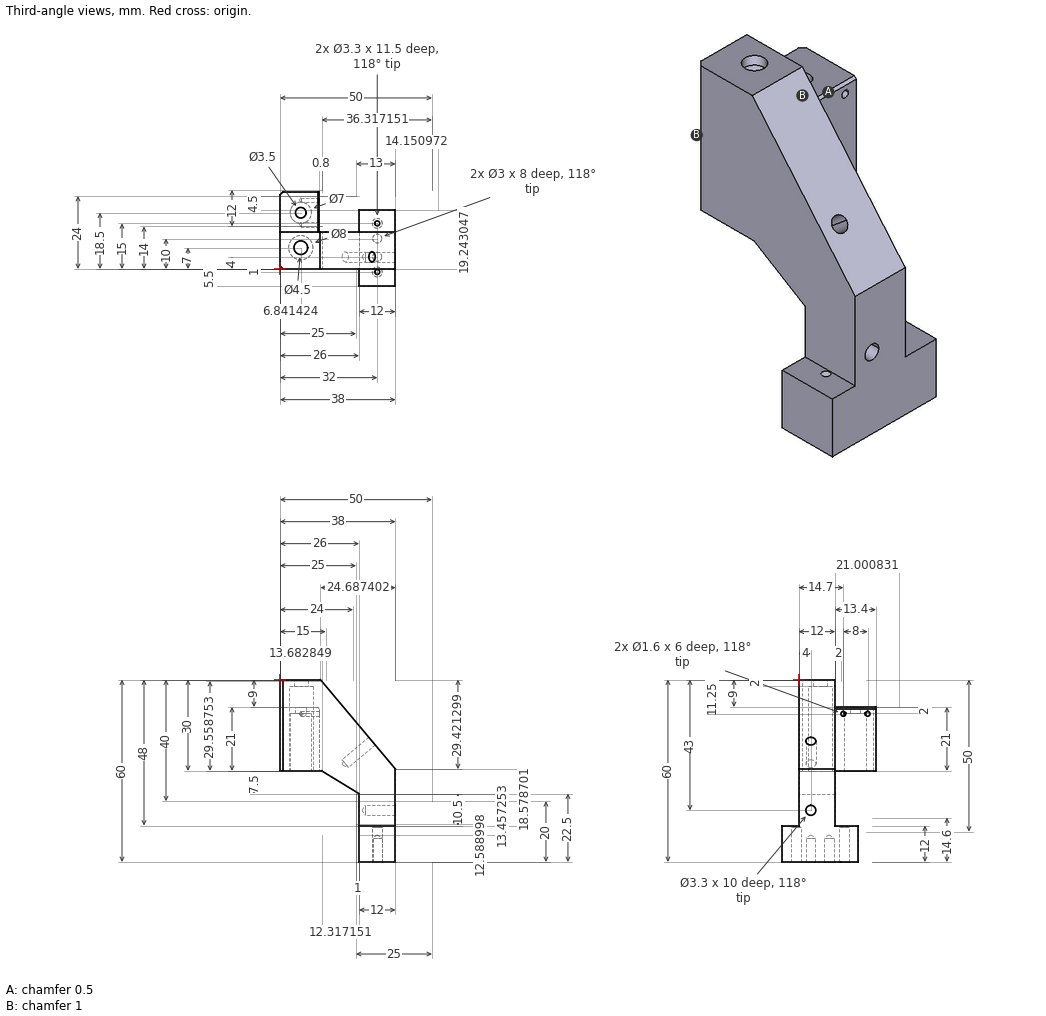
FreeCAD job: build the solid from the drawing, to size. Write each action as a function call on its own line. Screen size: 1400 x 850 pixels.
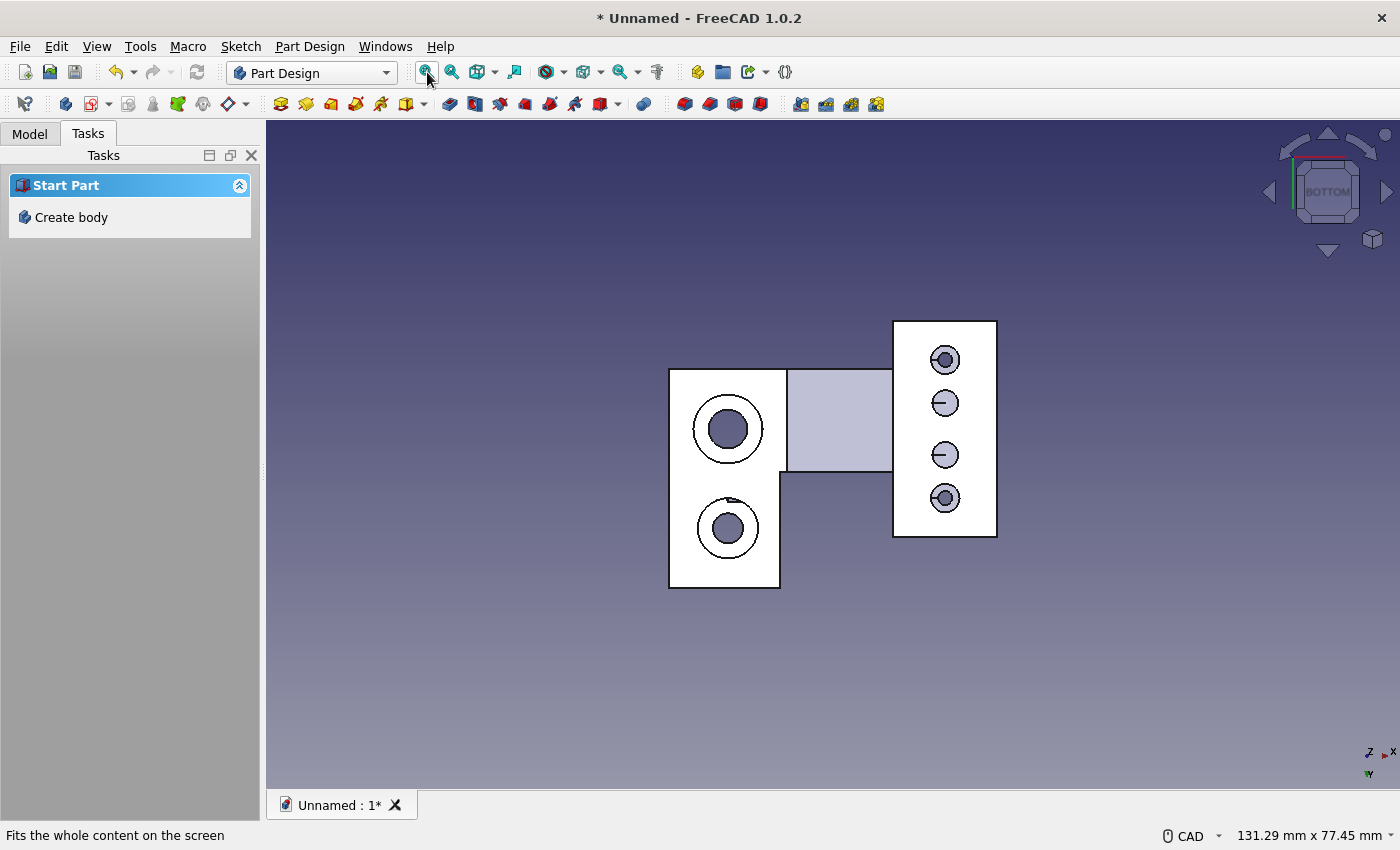
key(0)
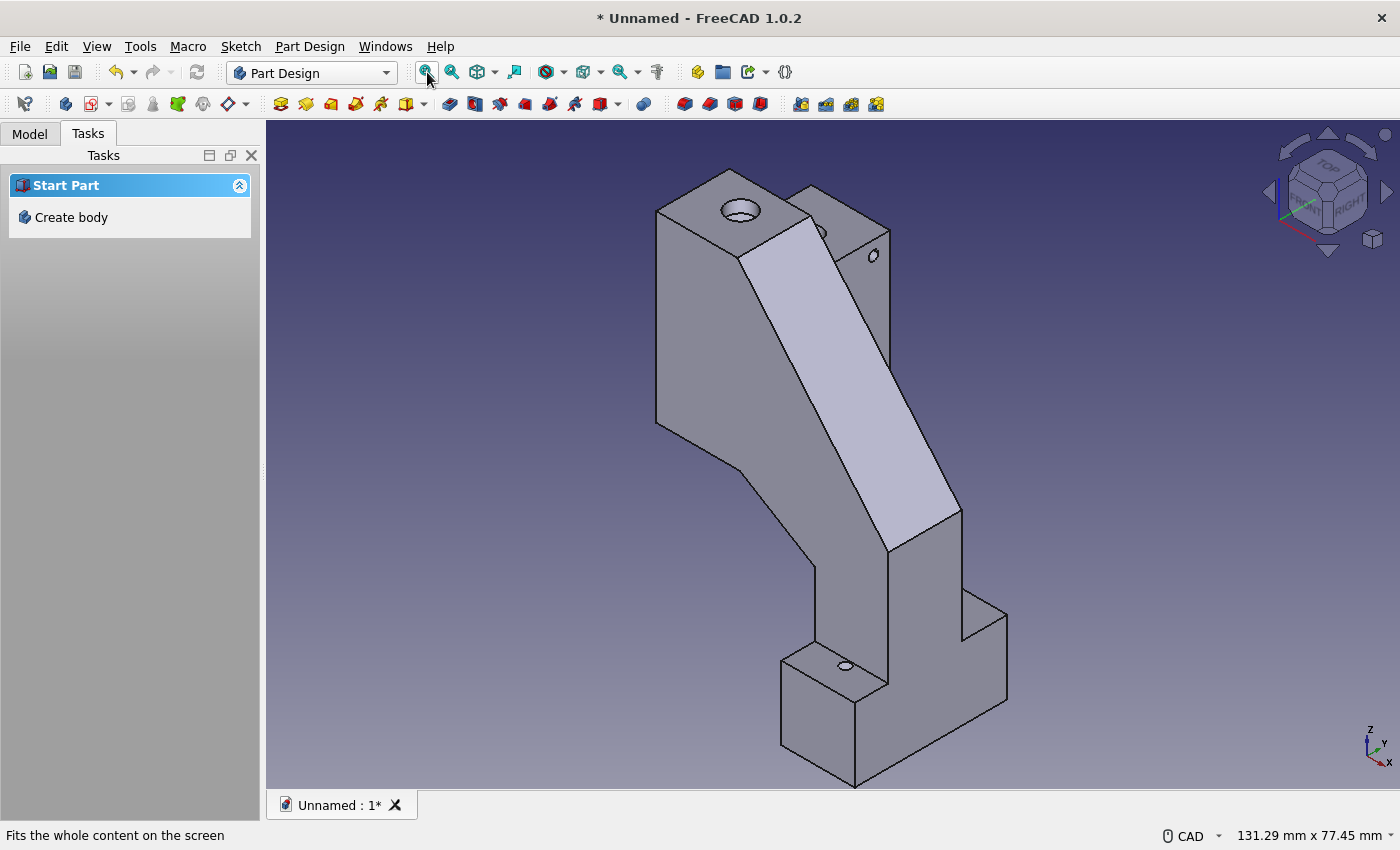
click(849, 253)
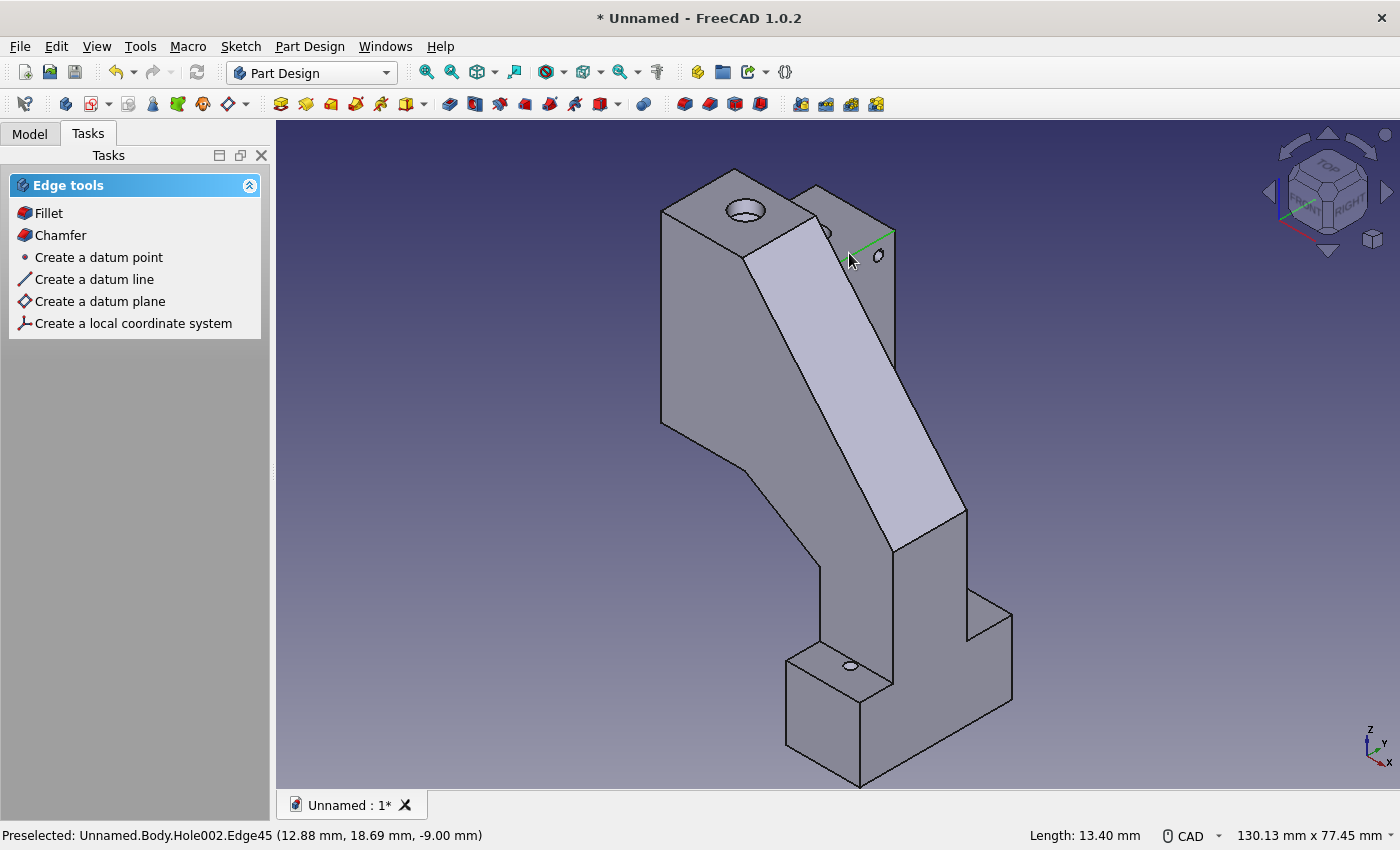
click(710, 104)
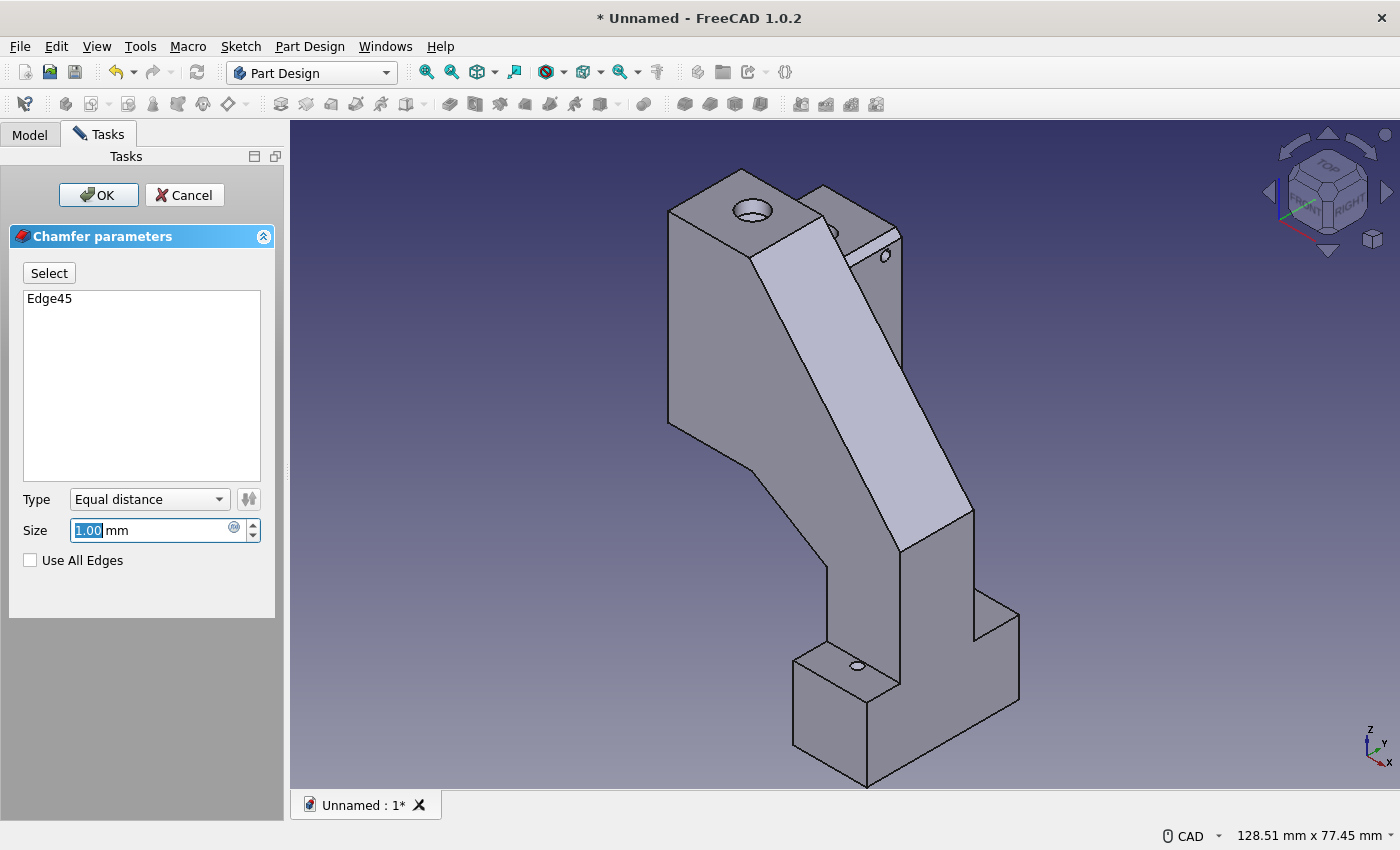
text(0.5)
key(Tab)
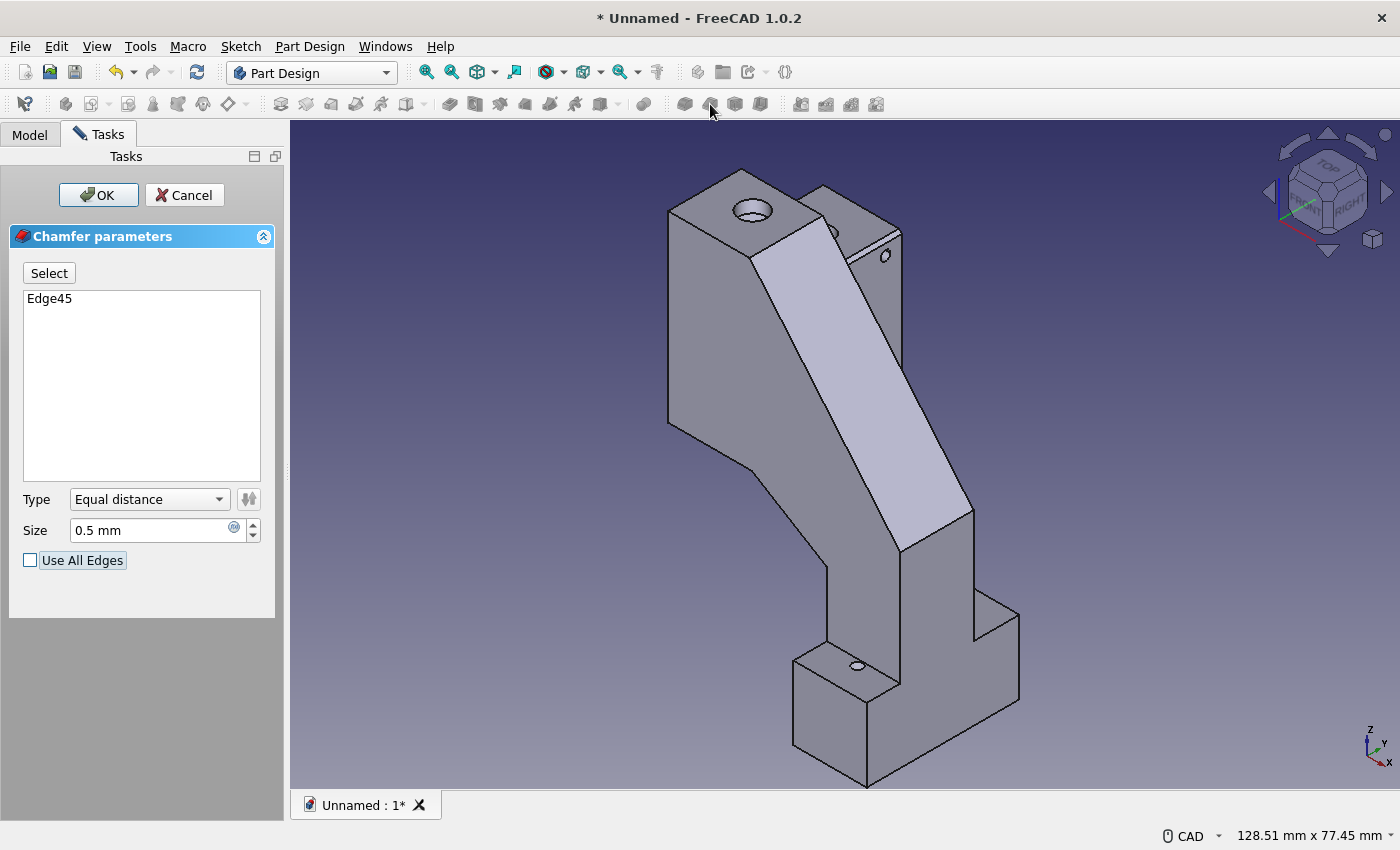
click(99, 195)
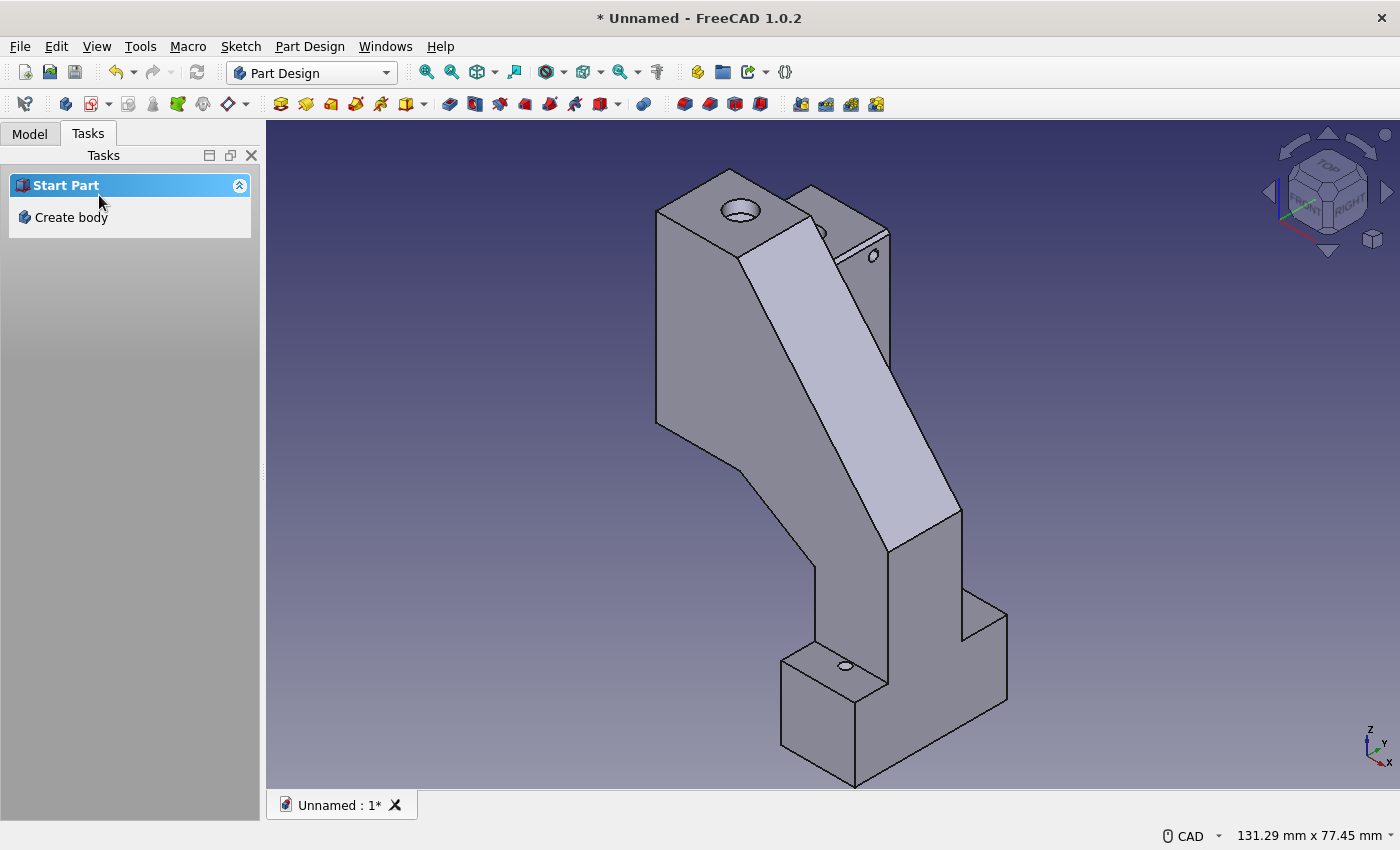
click(931, 696)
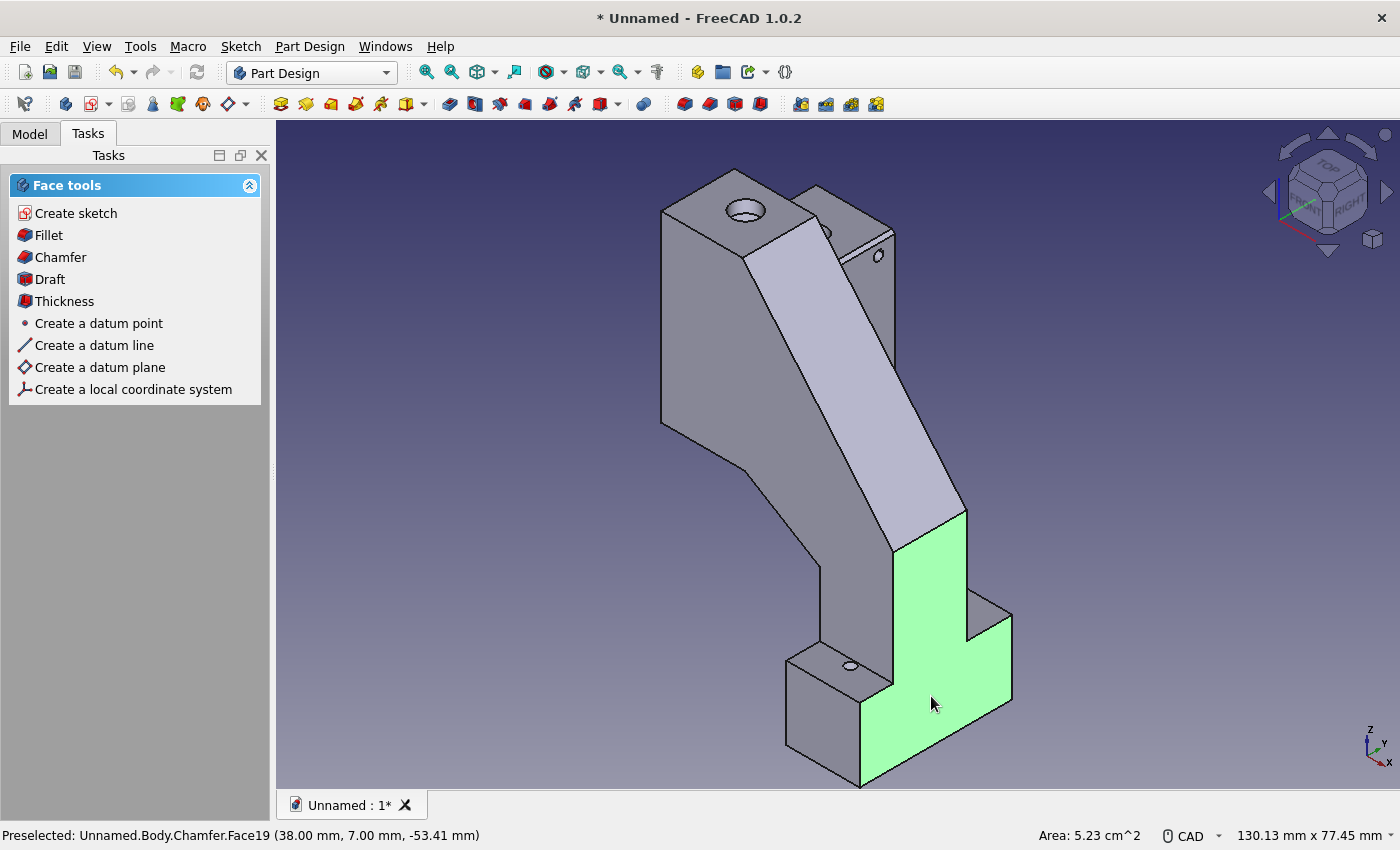
click(90, 104)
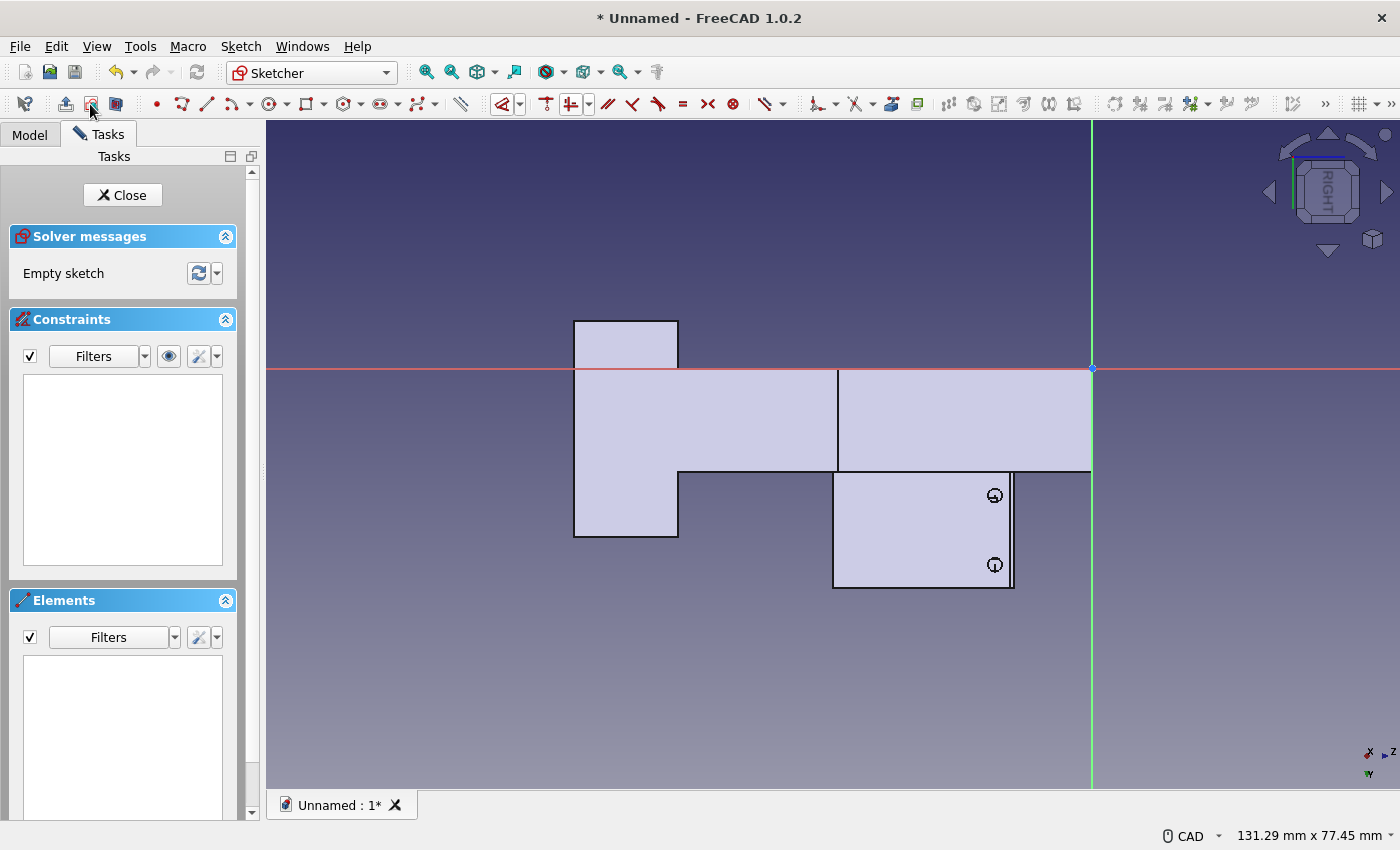
scroll(718, 400, up, 14)